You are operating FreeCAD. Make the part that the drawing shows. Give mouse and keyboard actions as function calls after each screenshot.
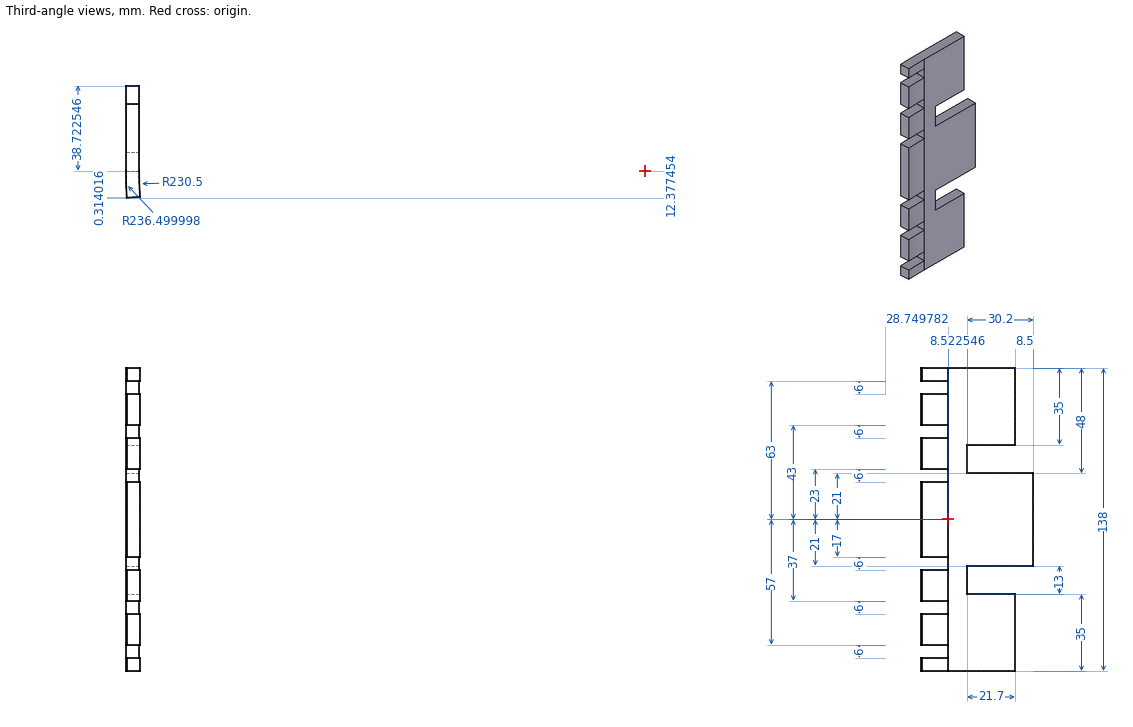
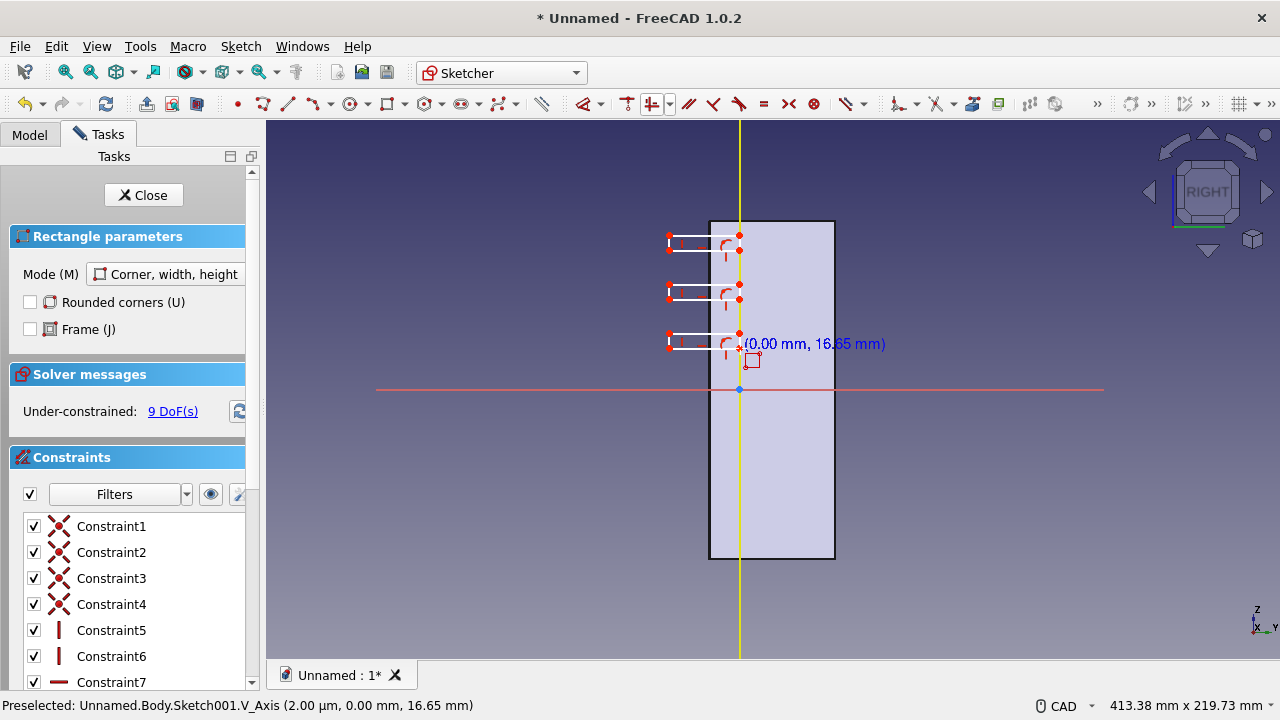
click(669, 432)
click(740, 446)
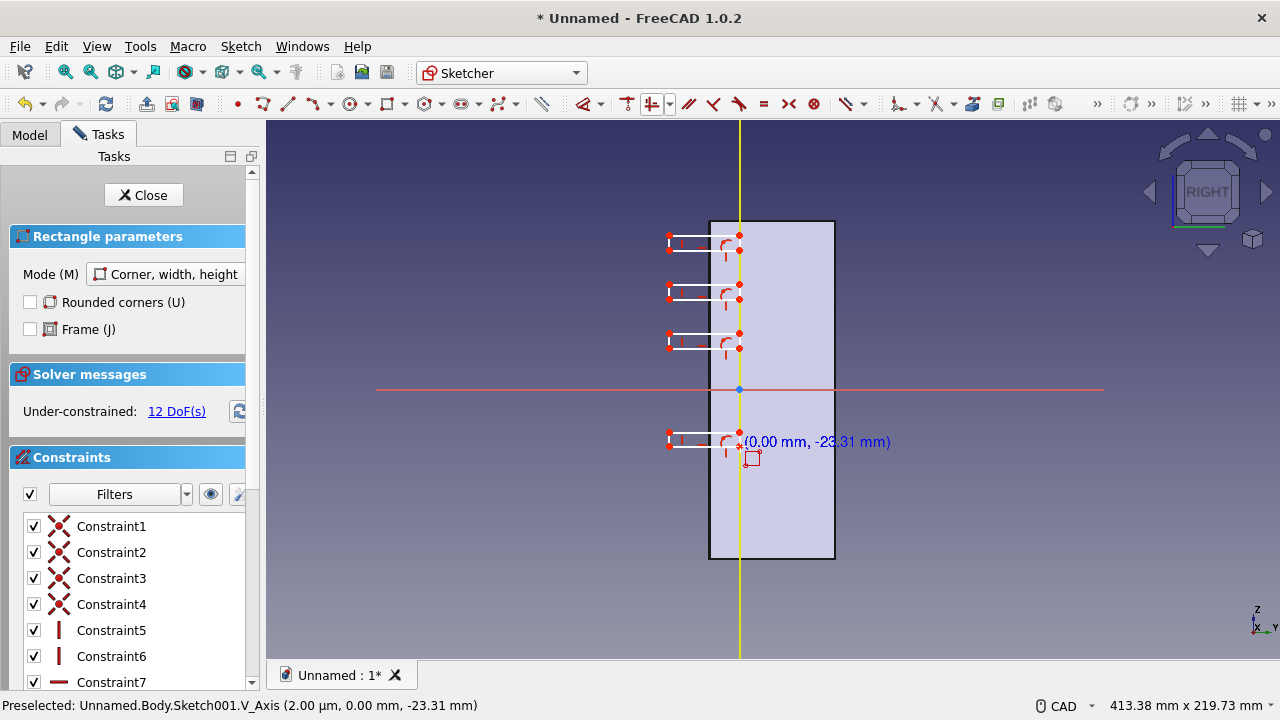
click(669, 481)
click(740, 495)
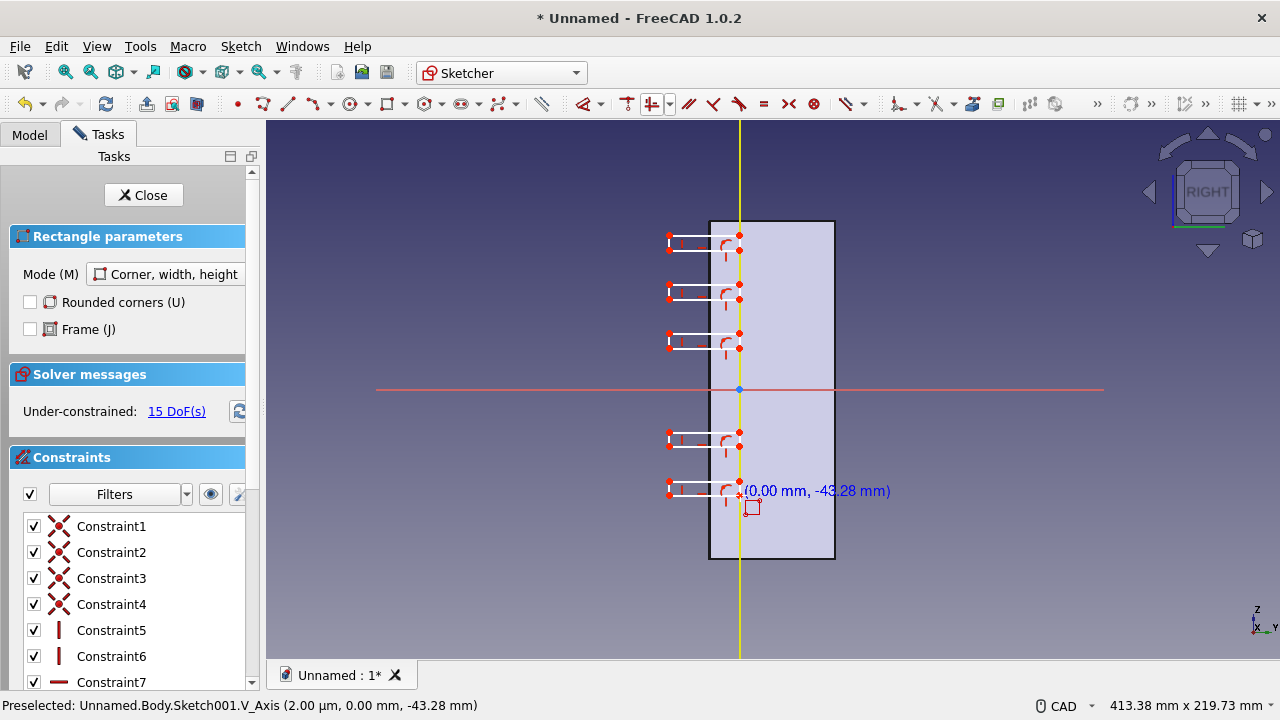
click(669, 530)
click(740, 544)
key(Escape)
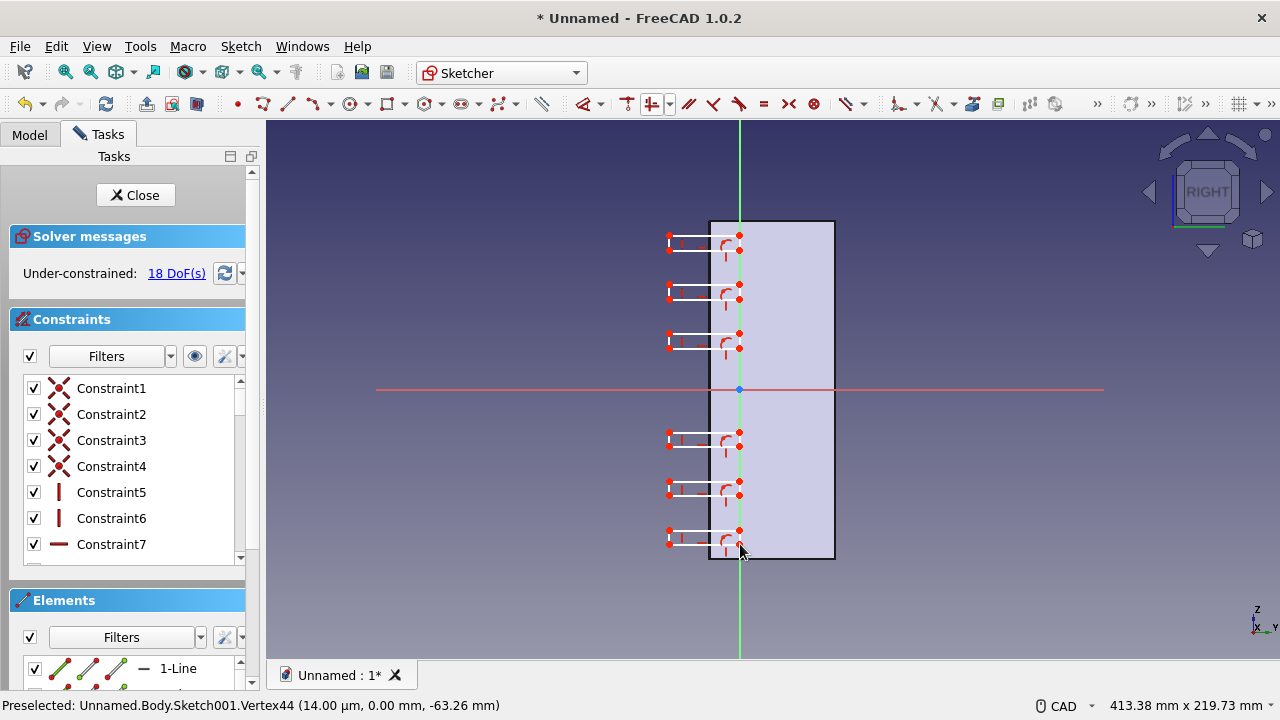
key(d)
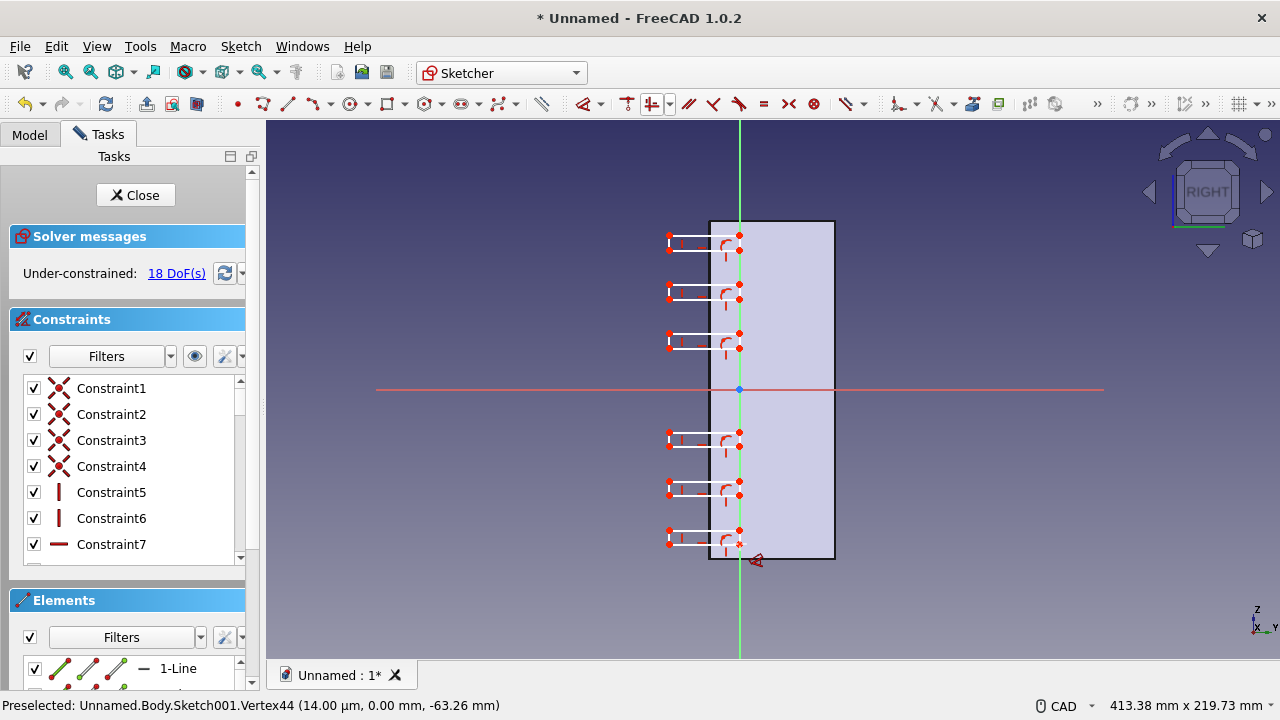
scroll(669, 243, up, 5)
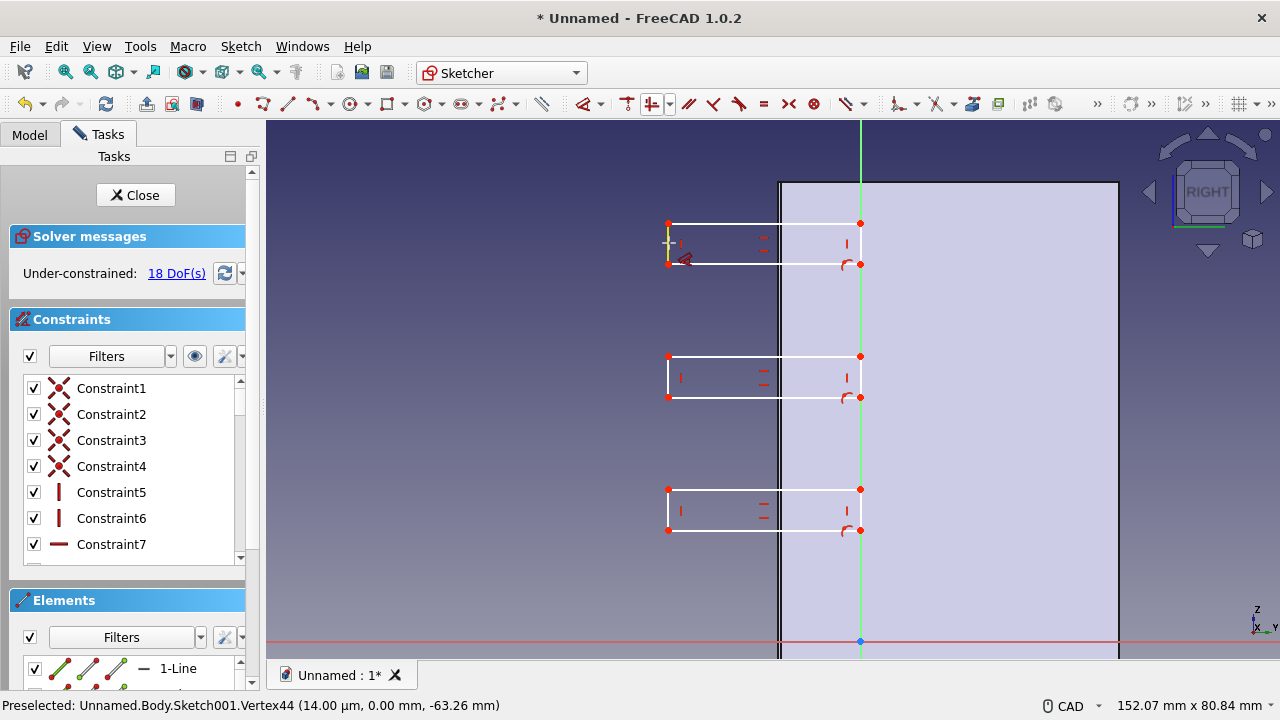
click(668, 244)
click(634, 244)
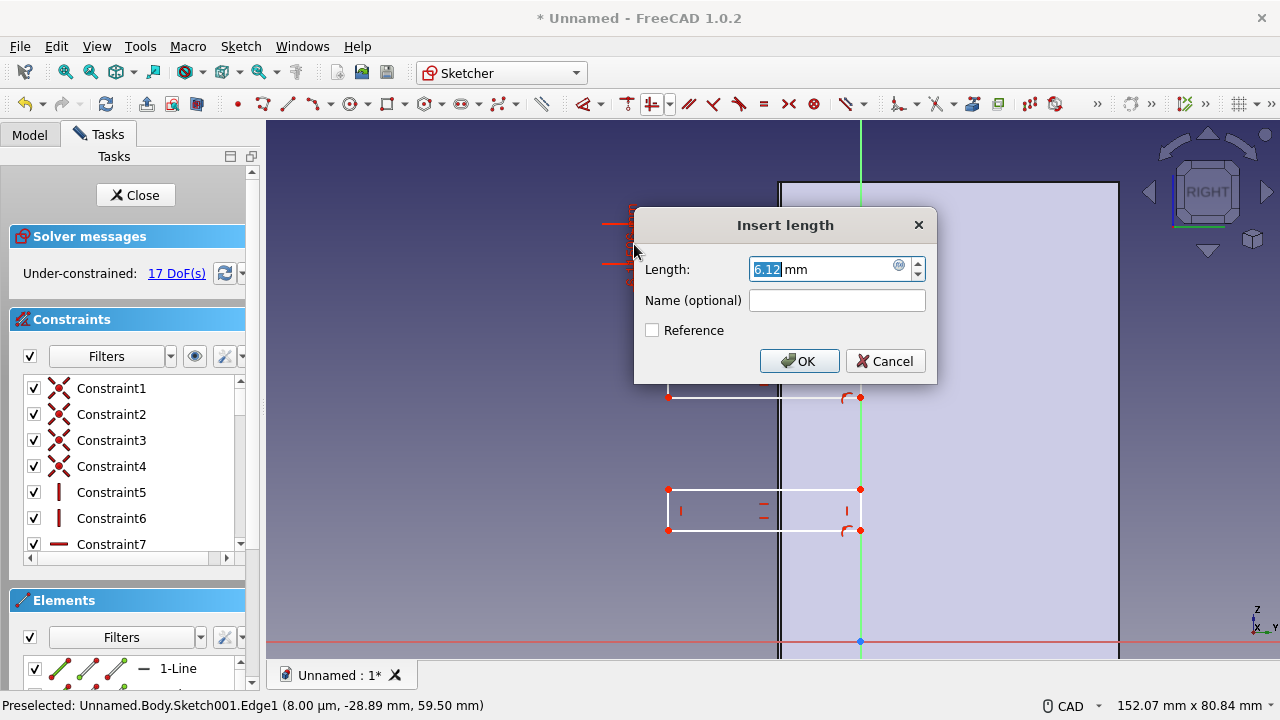
text(6)
key(Return)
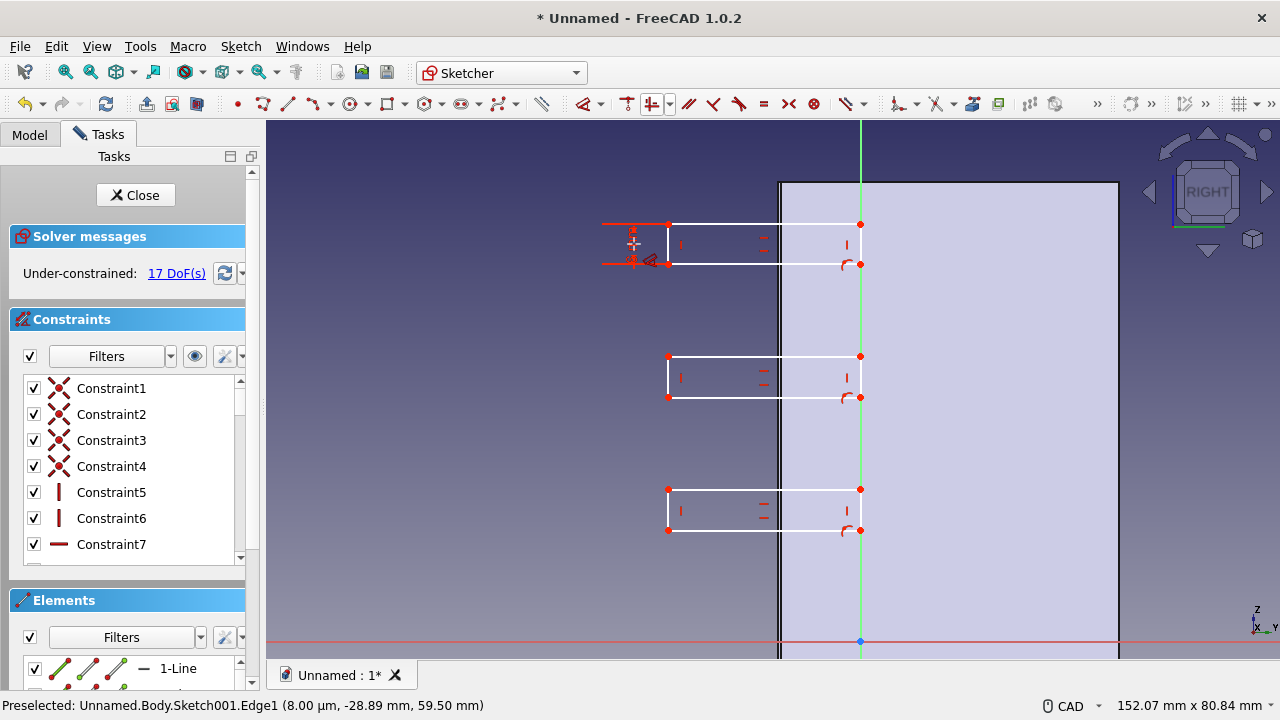
click(668, 369)
click(634, 377)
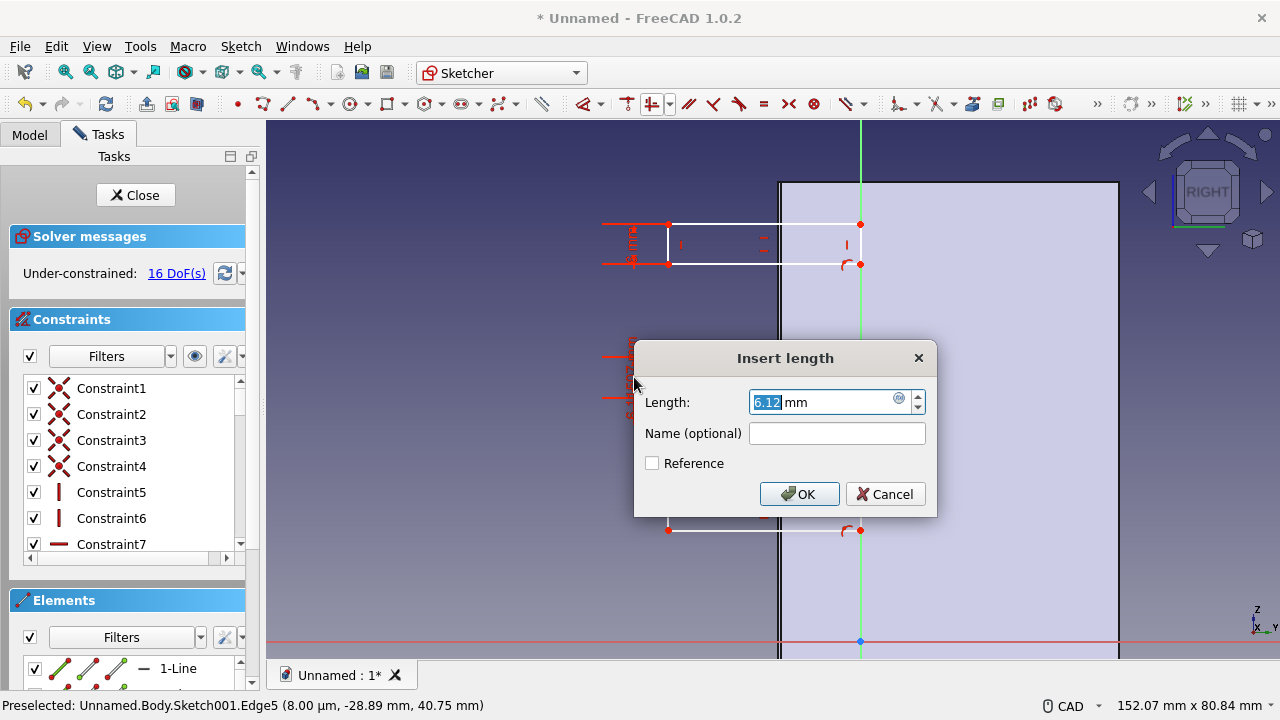
text(6)
key(Return)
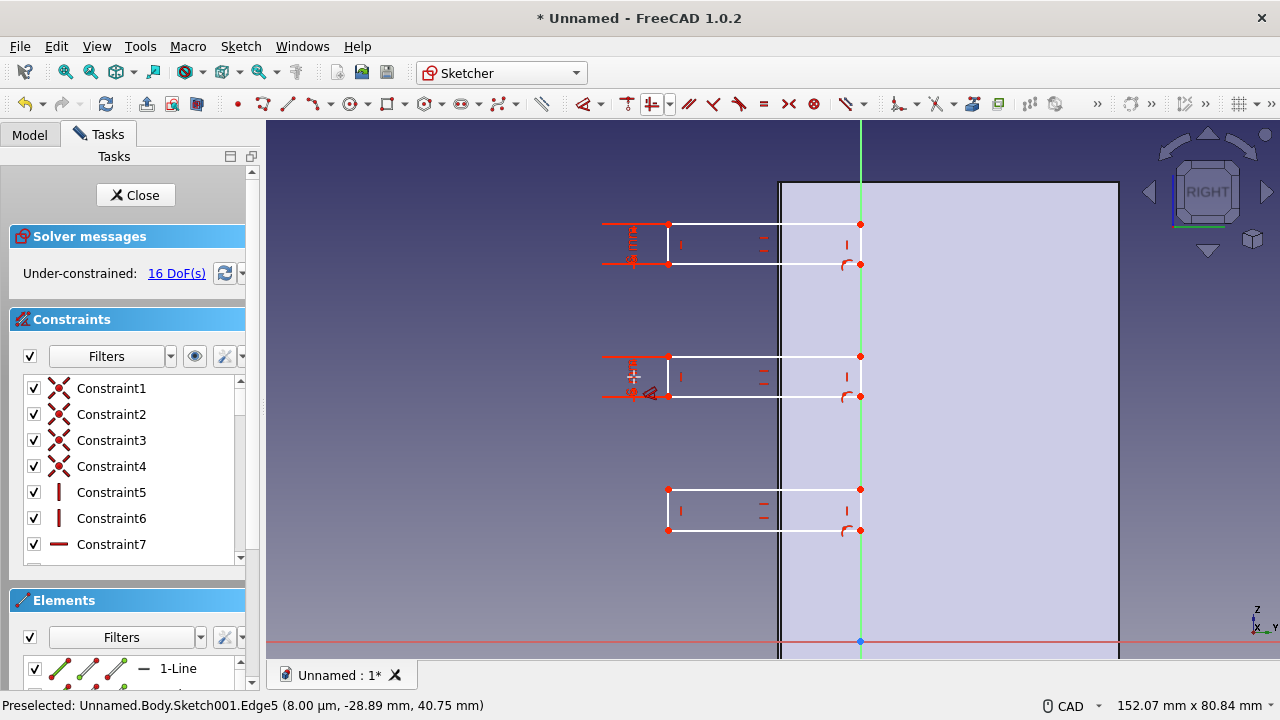
click(668, 502)
click(634, 510)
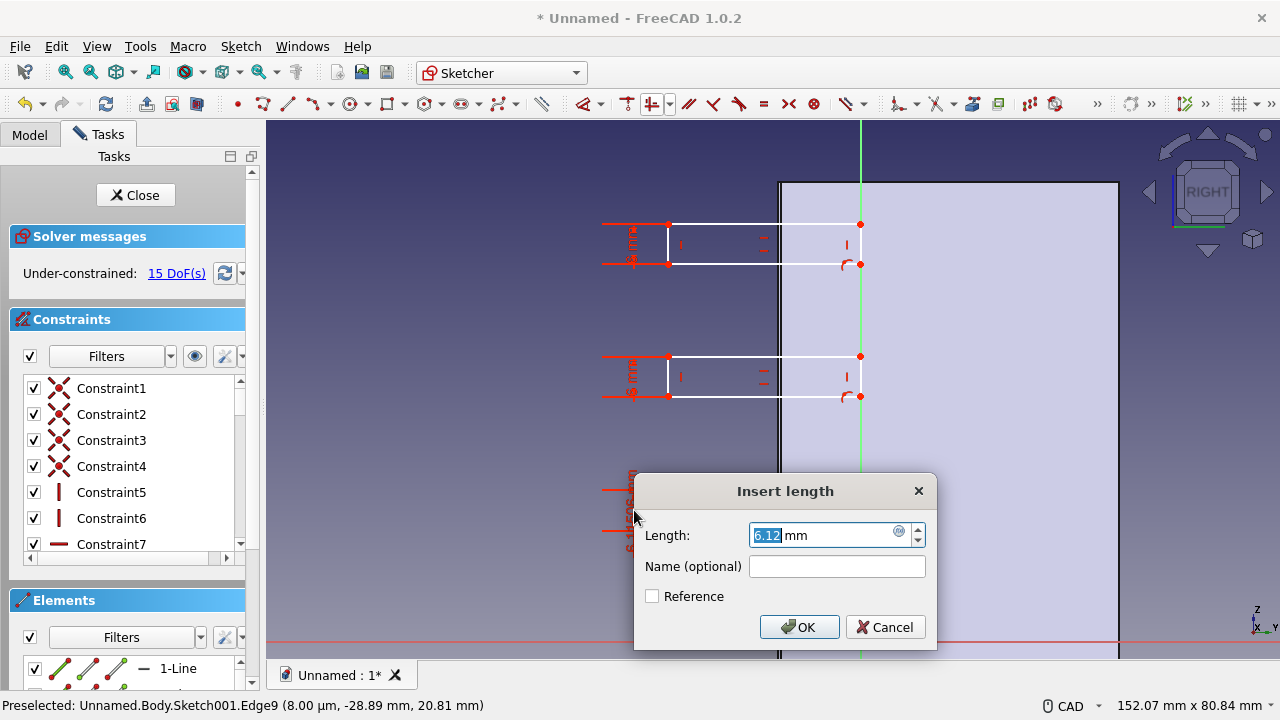
text(6)
key(Return)